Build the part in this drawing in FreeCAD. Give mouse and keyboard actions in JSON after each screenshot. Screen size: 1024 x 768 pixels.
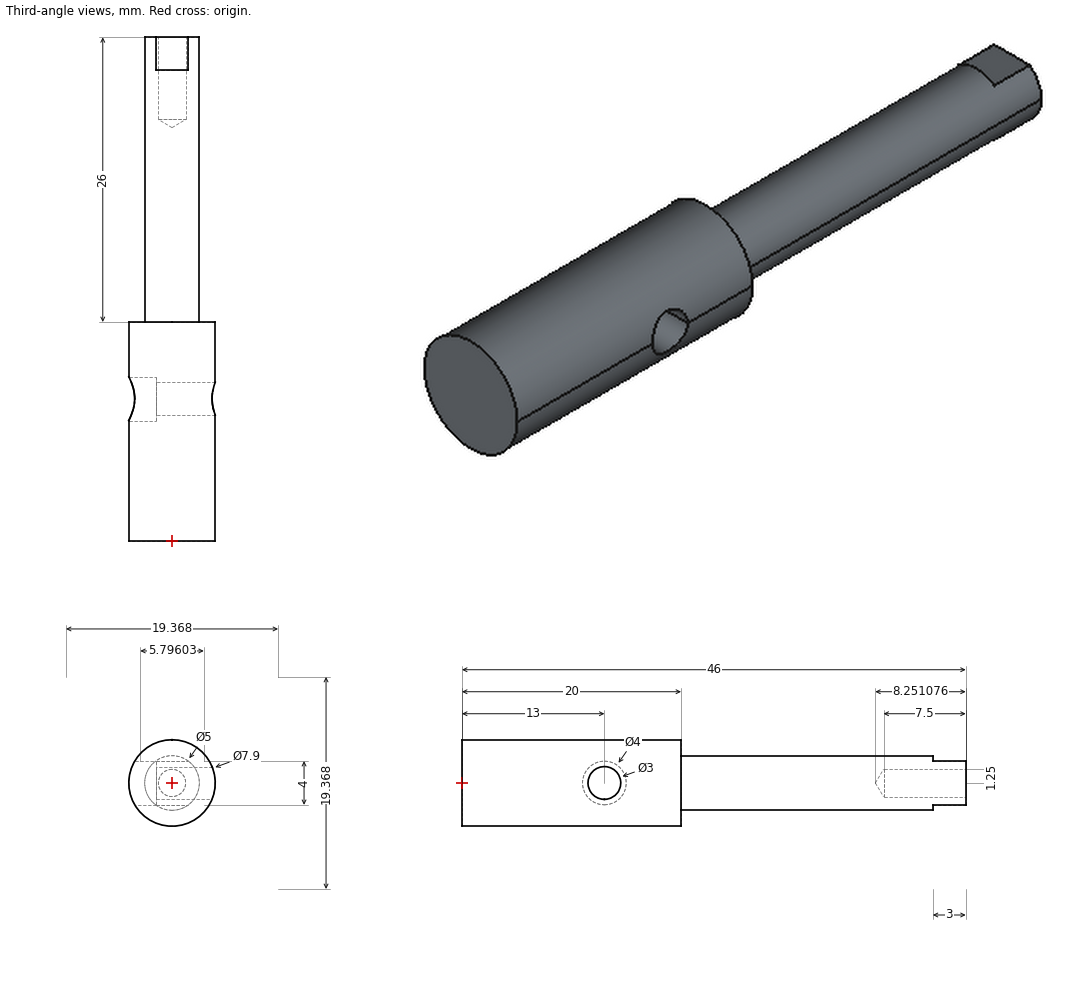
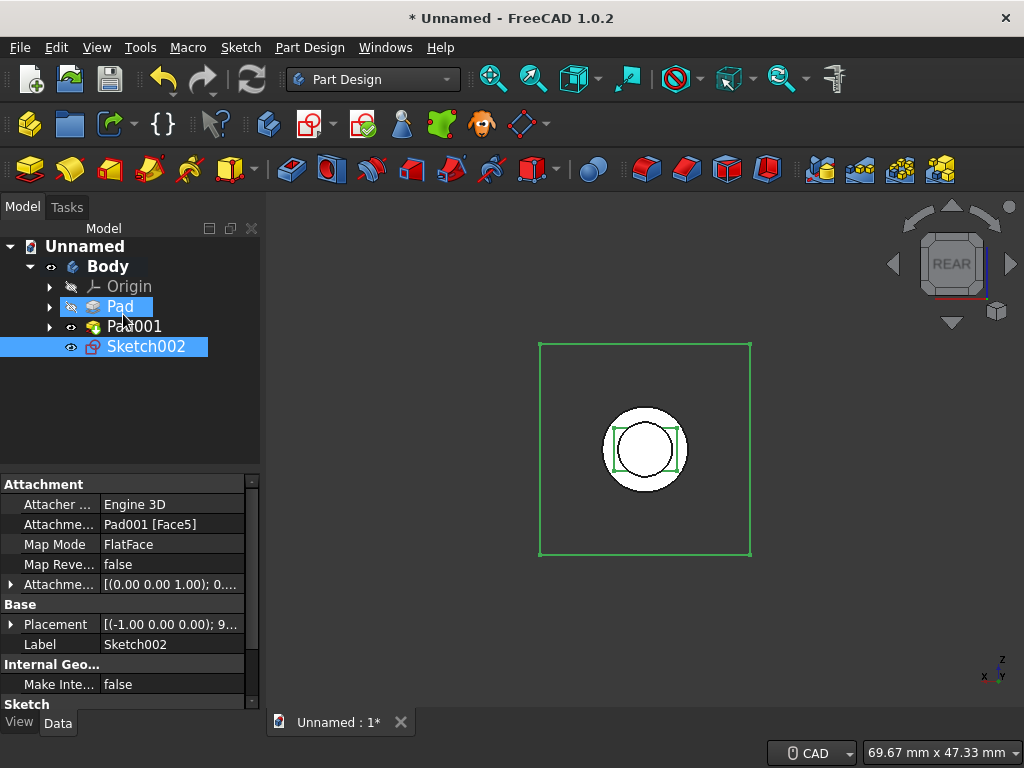
{"action": "left_click", "coordinate": [292, 170]}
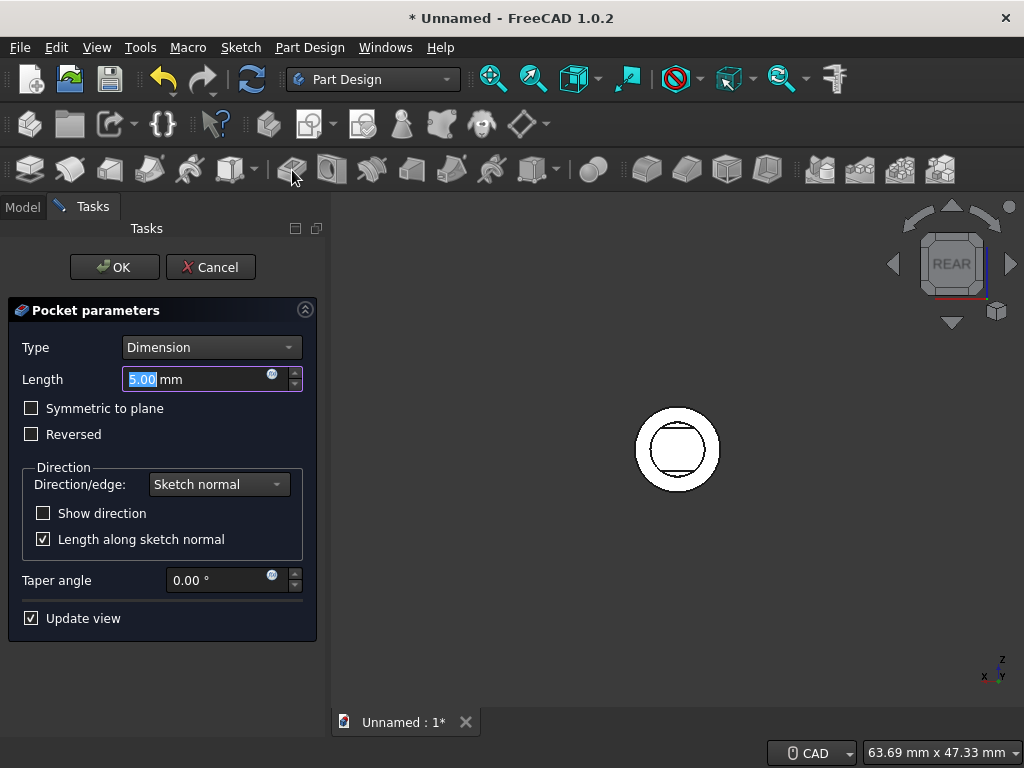
{"action": "type", "text": "3"}
{"action": "key", "text": "Tab"}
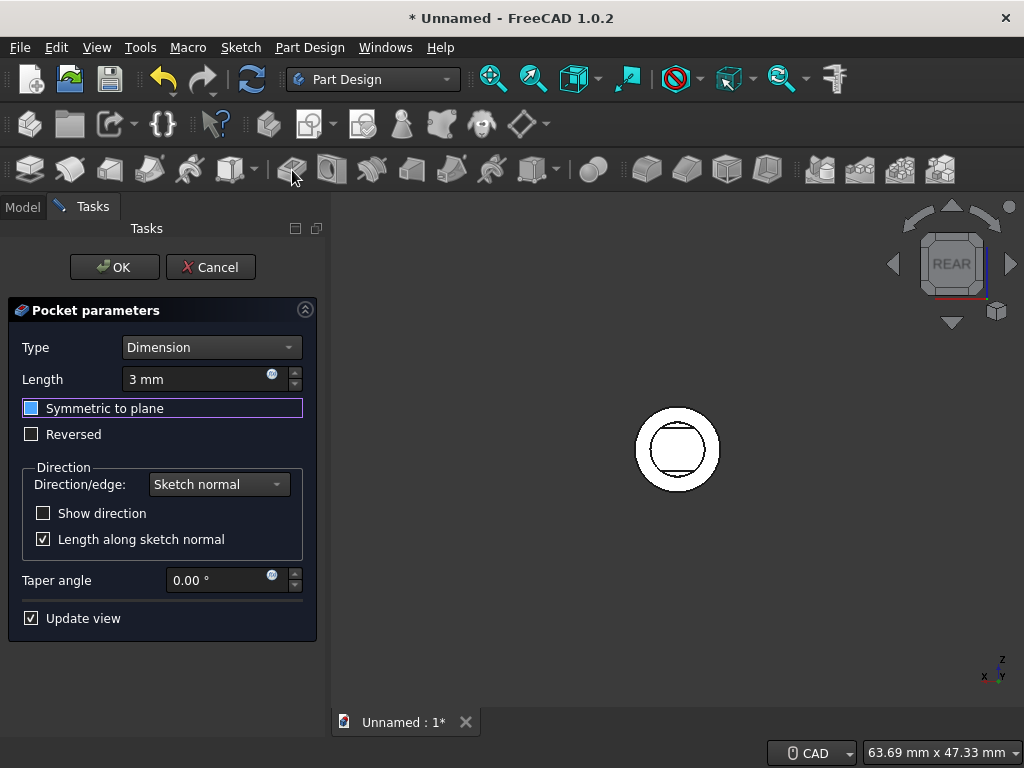
{"action": "left_click", "coordinate": [115, 267]}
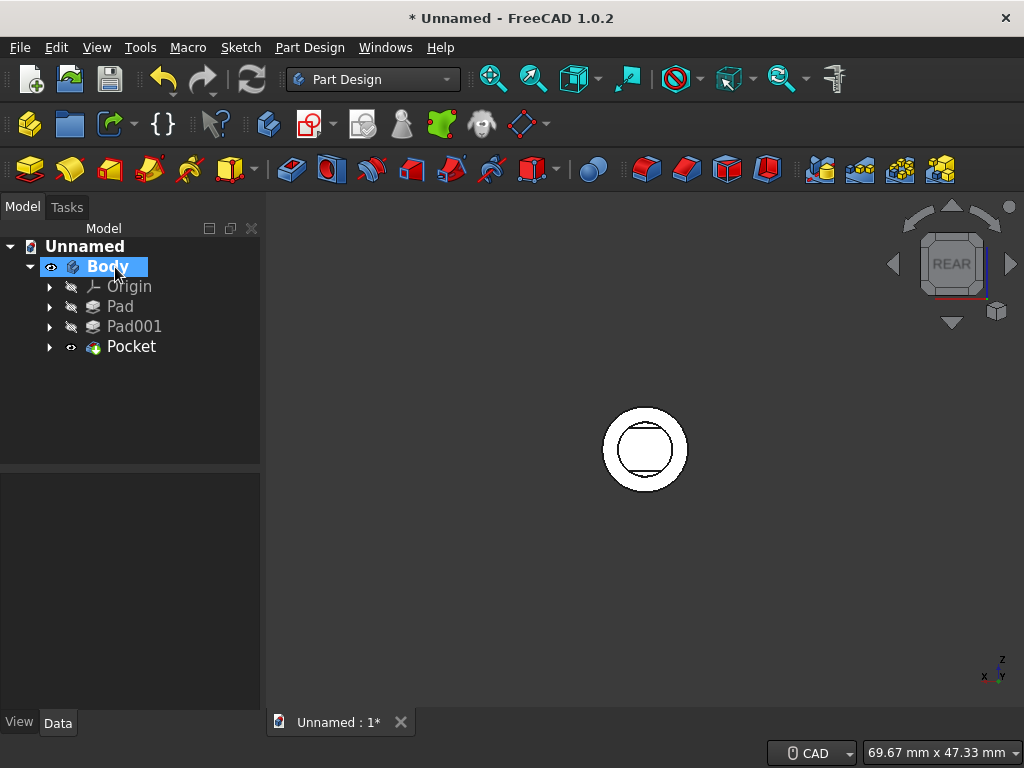
{"action": "left_click", "coordinate": [494, 80]}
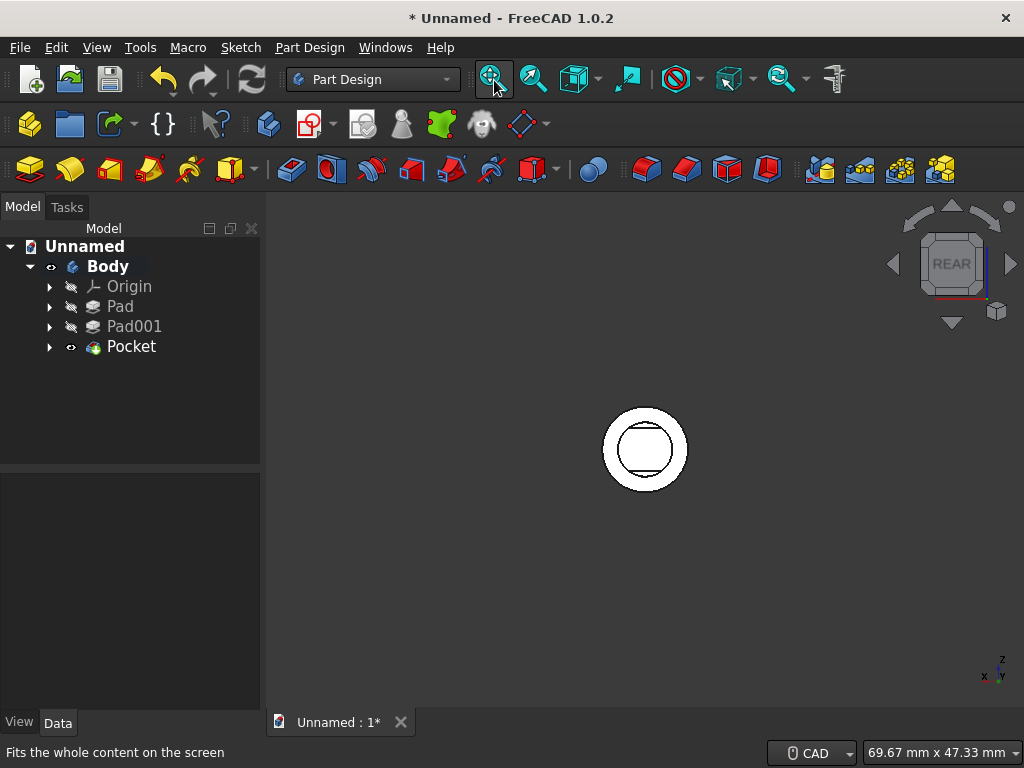
{"action": "left_click", "coordinate": [310, 124]}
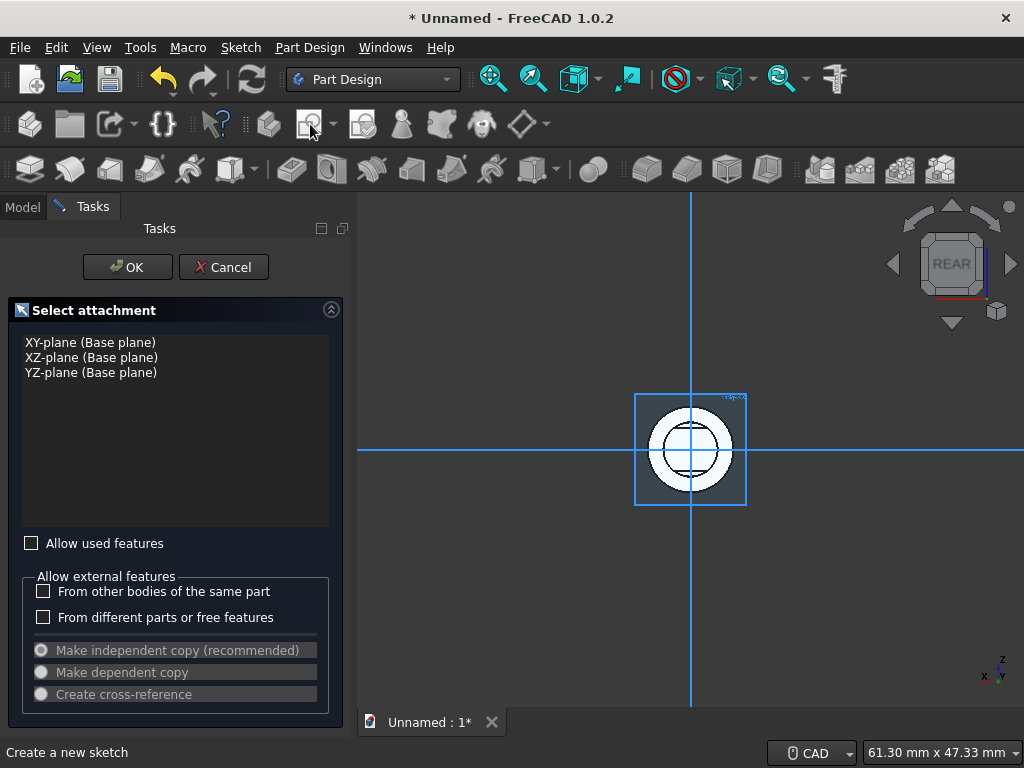
{"action": "left_click", "coordinate": [82, 372]}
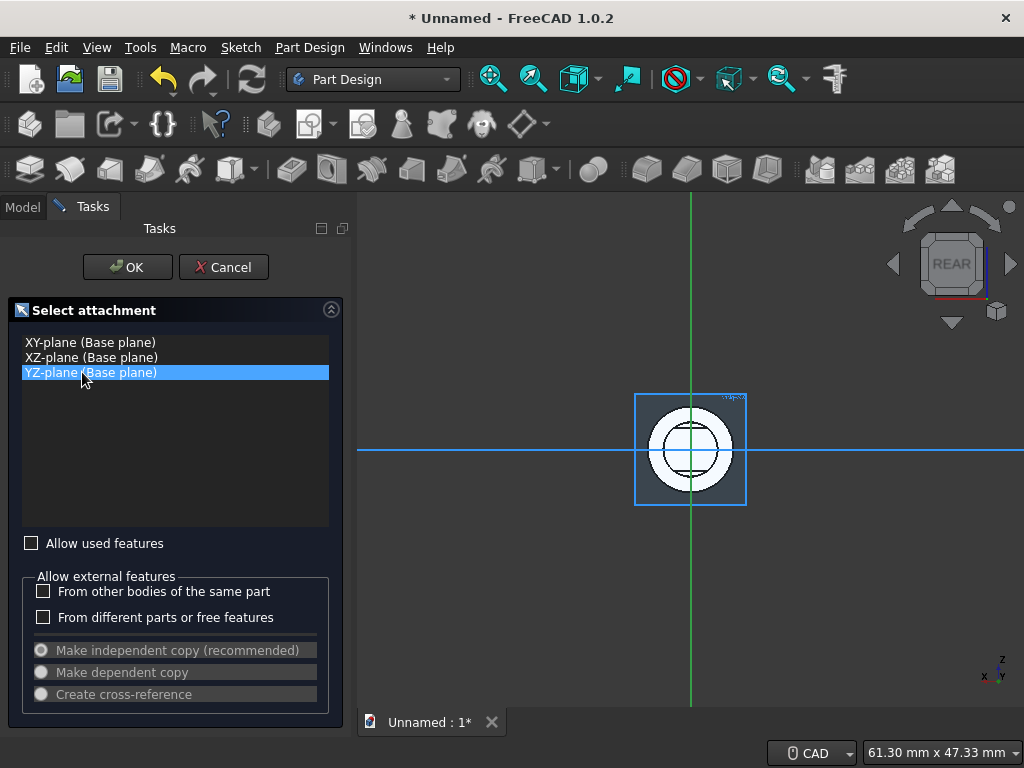
{"action": "left_click", "coordinate": [128, 267]}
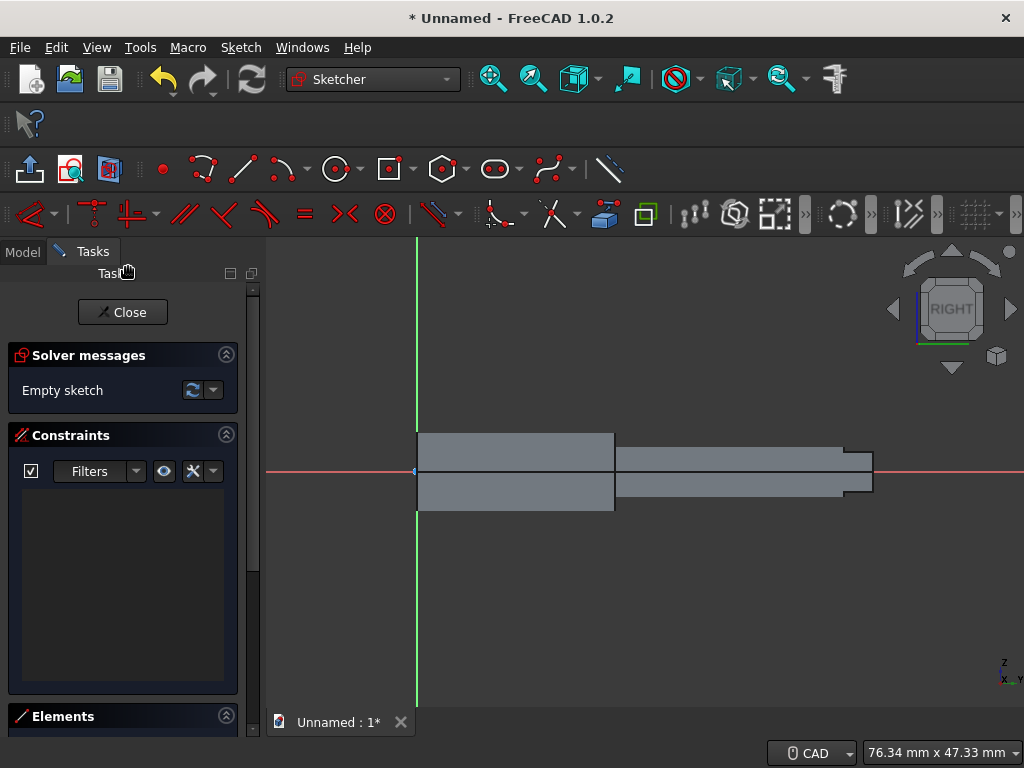
{"action": "left_click", "coordinate": [110, 170]}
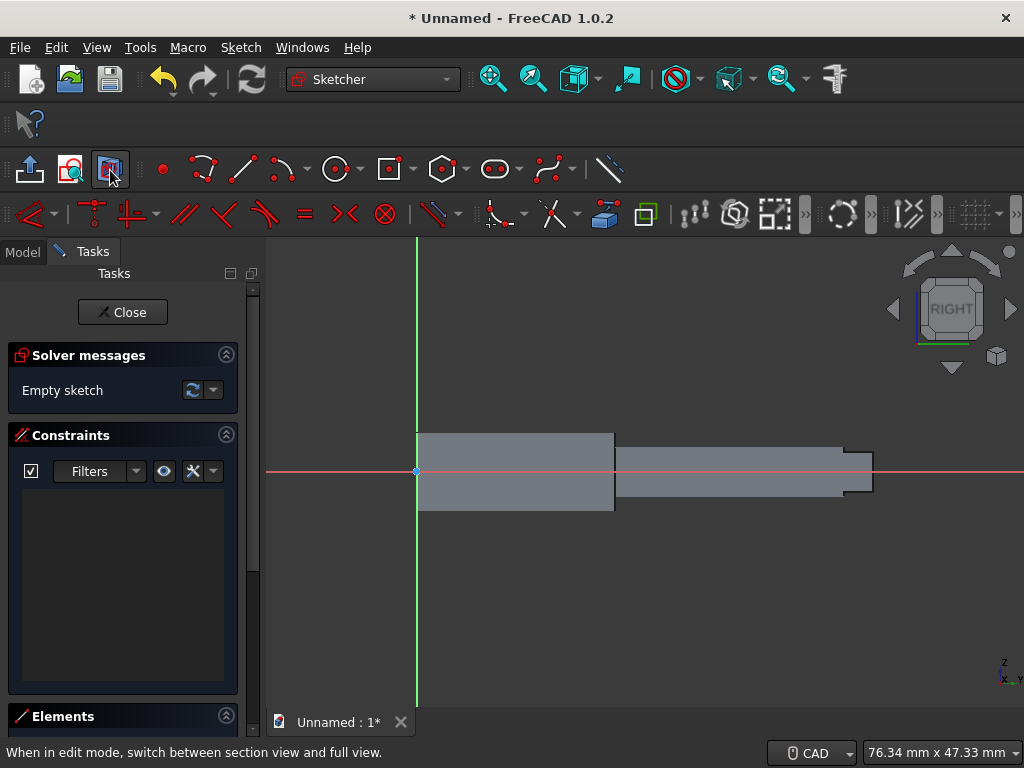
{"action": "scroll", "coordinate": [542, 472], "scroll_direction": "up", "scroll_amount": 11}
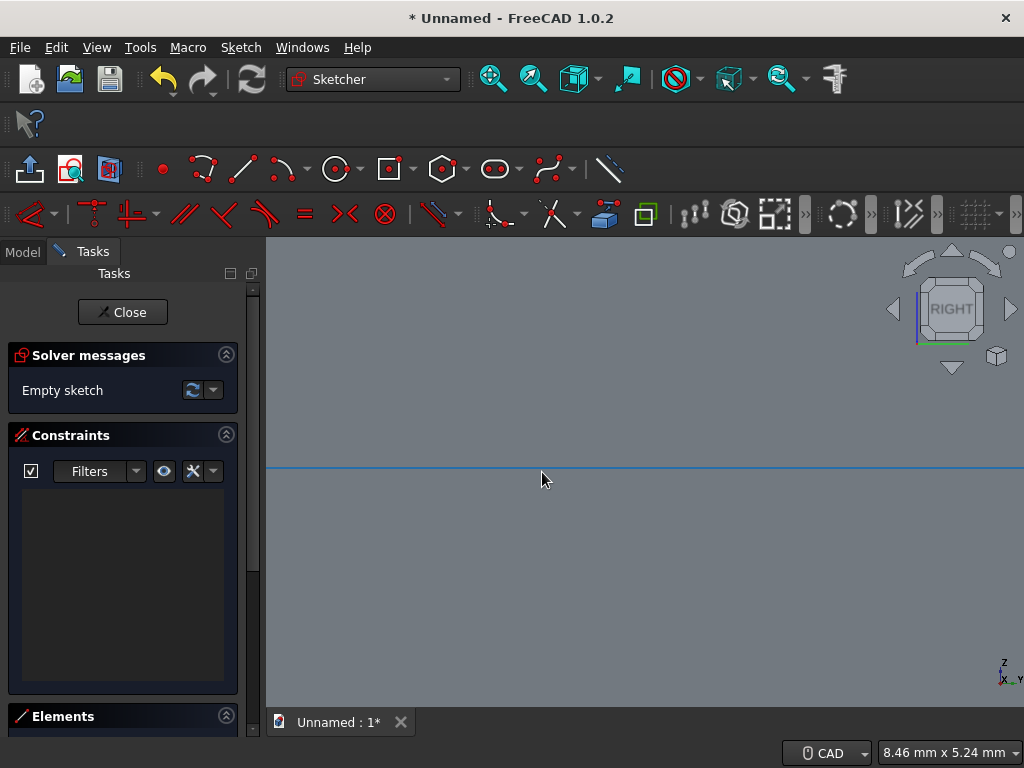
{"action": "left_click", "coordinate": [336, 170]}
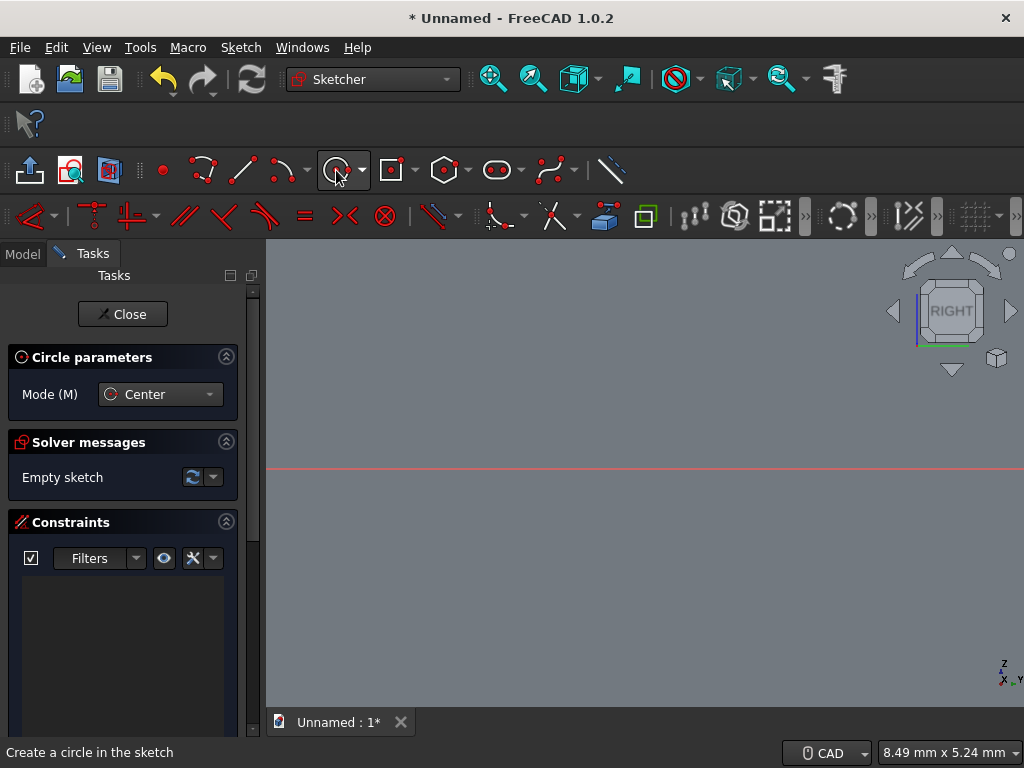
{"action": "left_click", "coordinate": [573, 469]}
{"action": "mouse_move", "coordinate": [667, 374]}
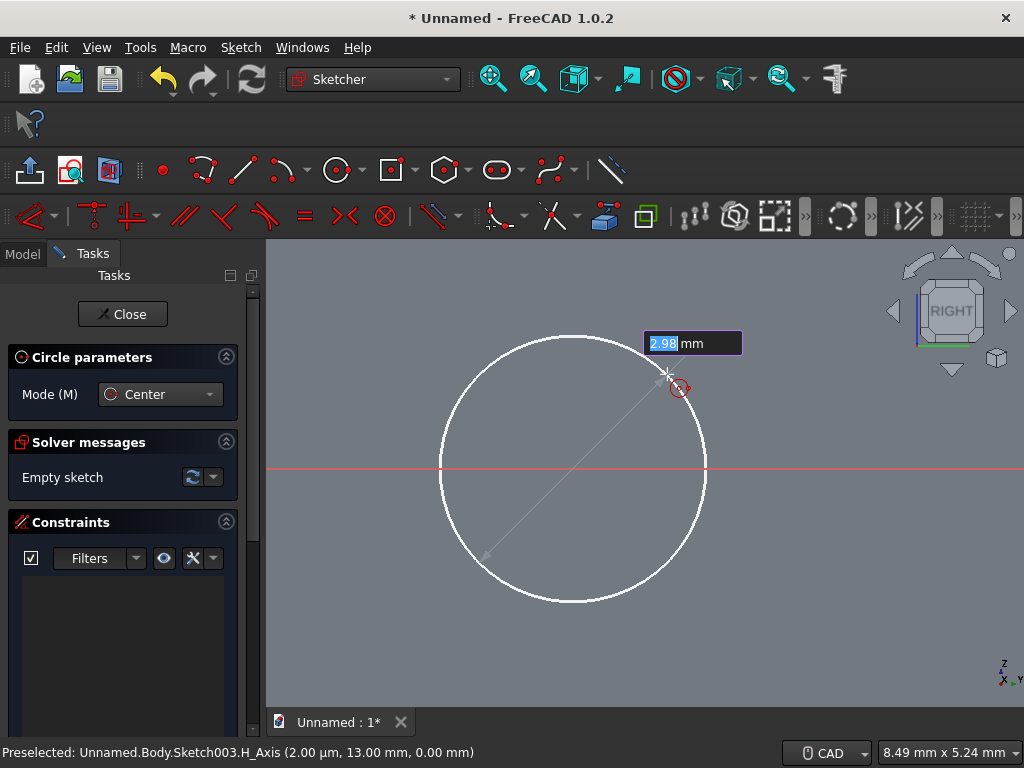
{"action": "type", "text": "3"}
{"action": "key", "text": "Return"}
{"action": "key", "text": "Escape"}